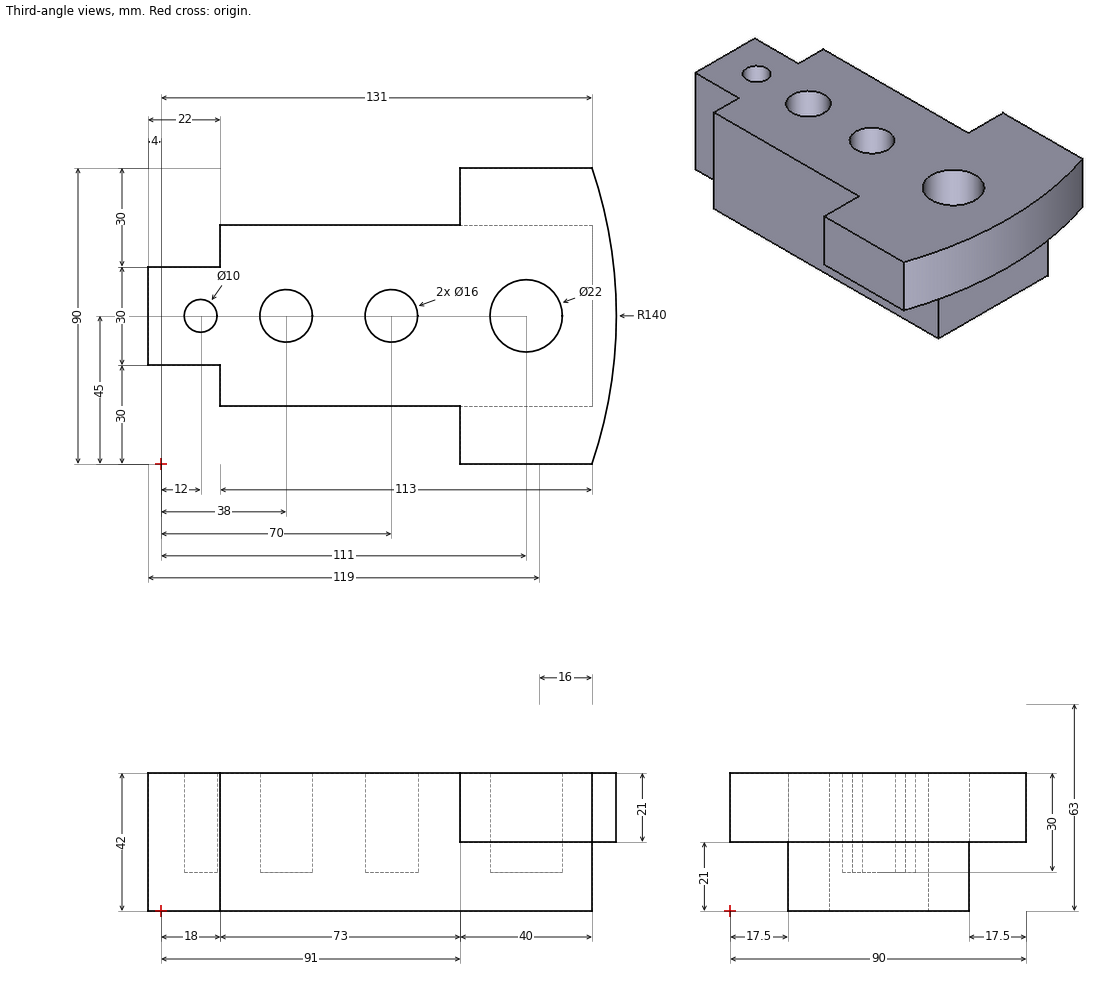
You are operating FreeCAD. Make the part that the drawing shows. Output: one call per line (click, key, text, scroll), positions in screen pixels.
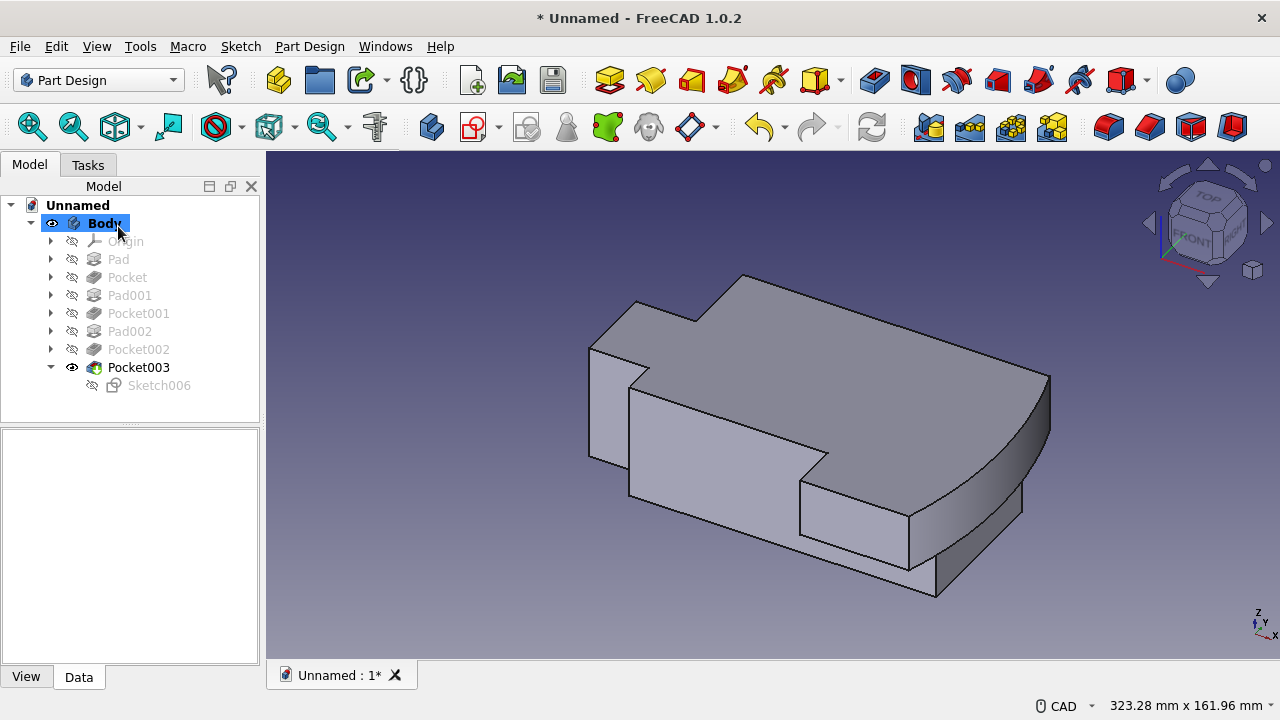
key(4)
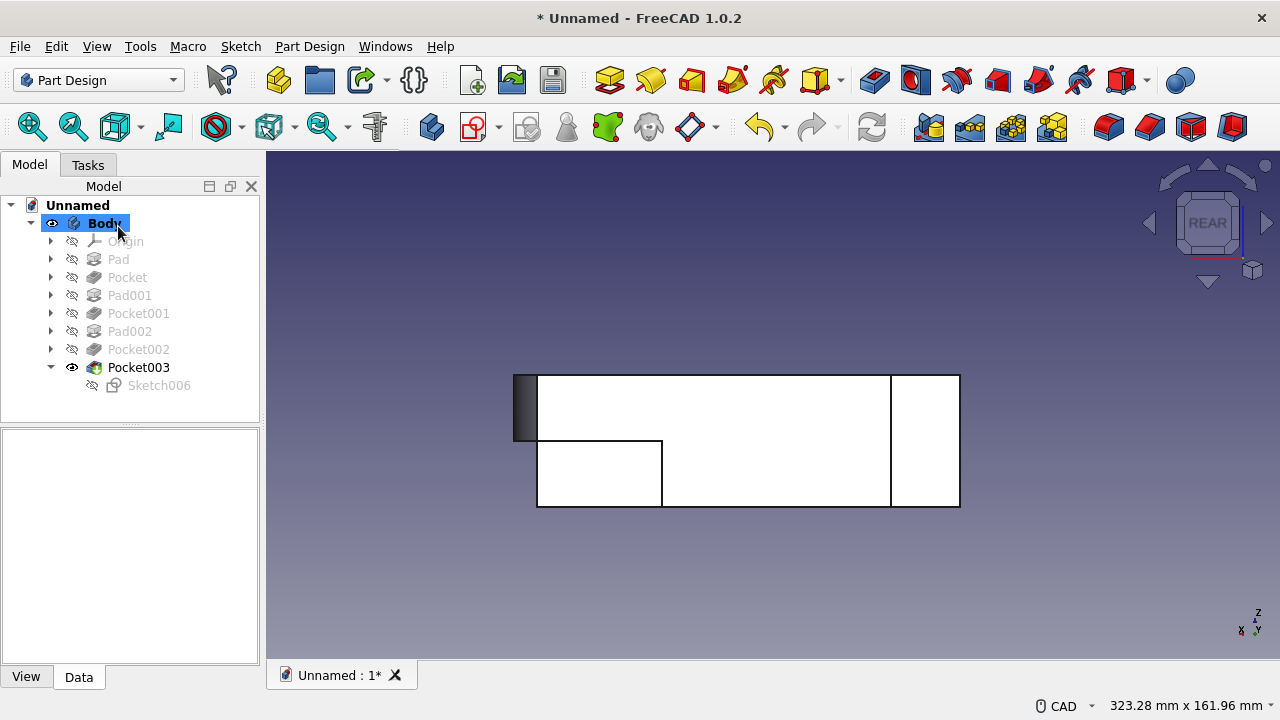
click(33, 128)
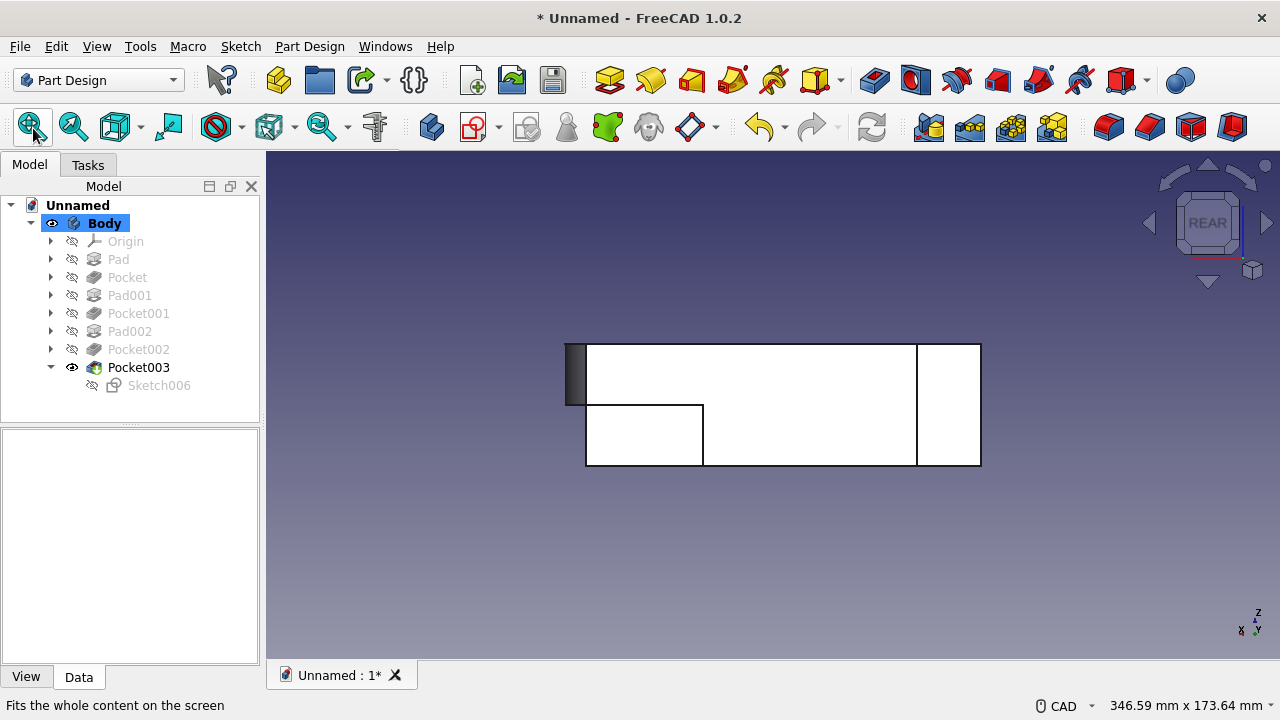
click(799, 404)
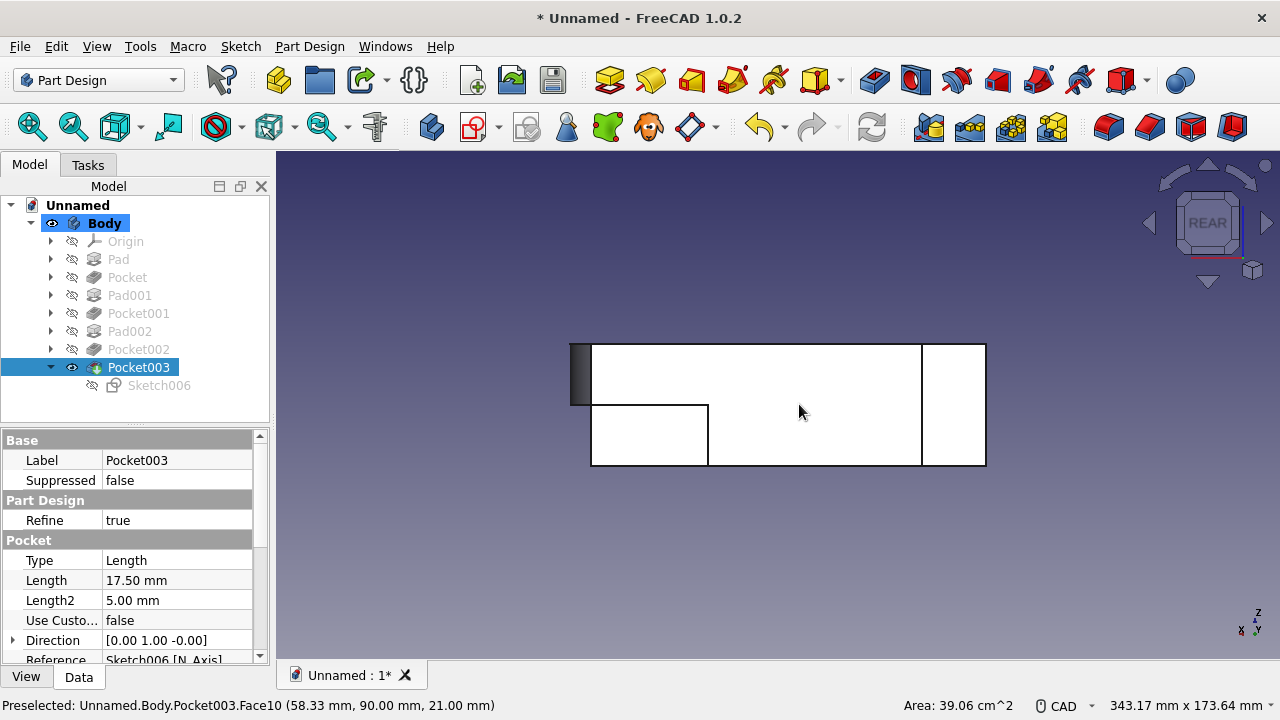
click(472, 128)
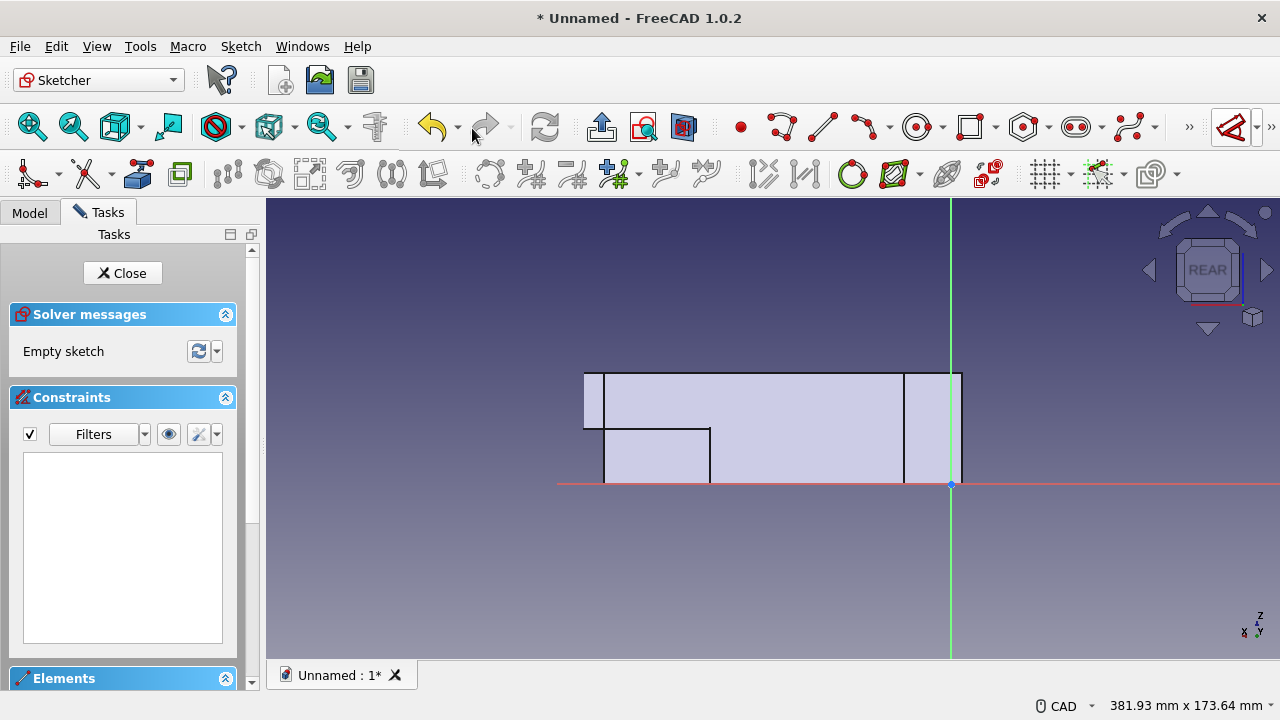
scroll(934, 428, up, 4)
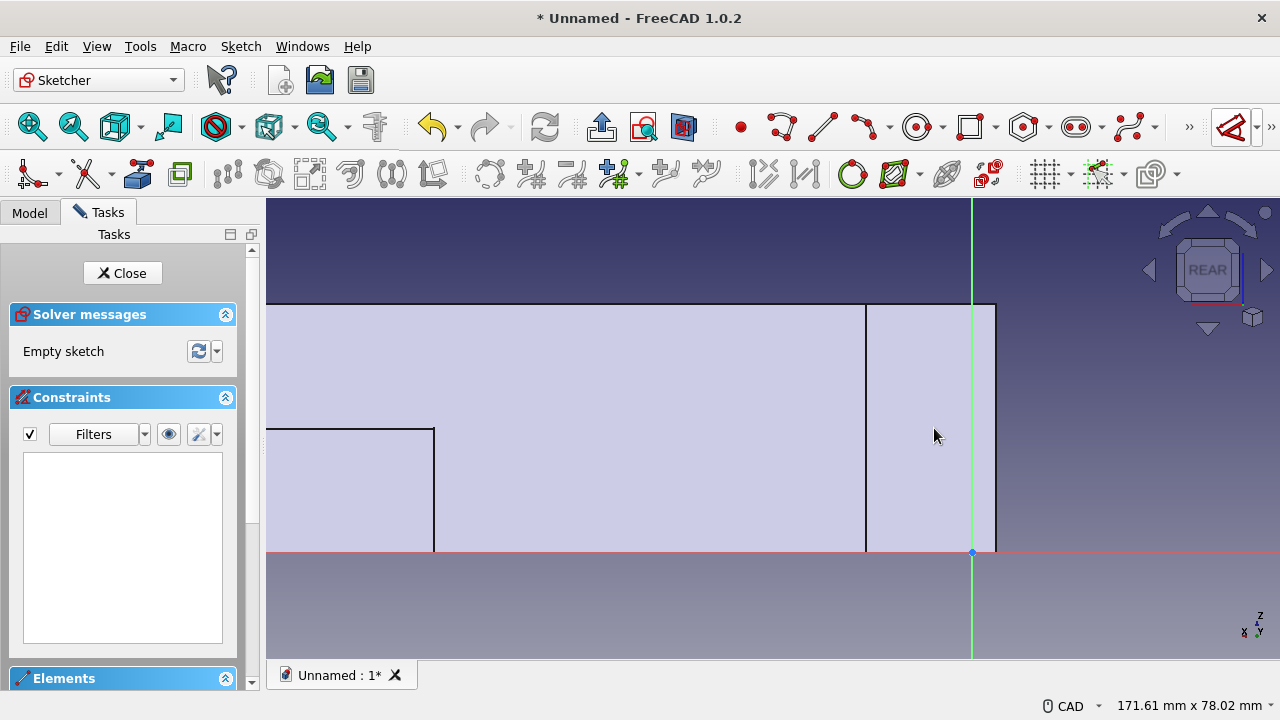
click(970, 128)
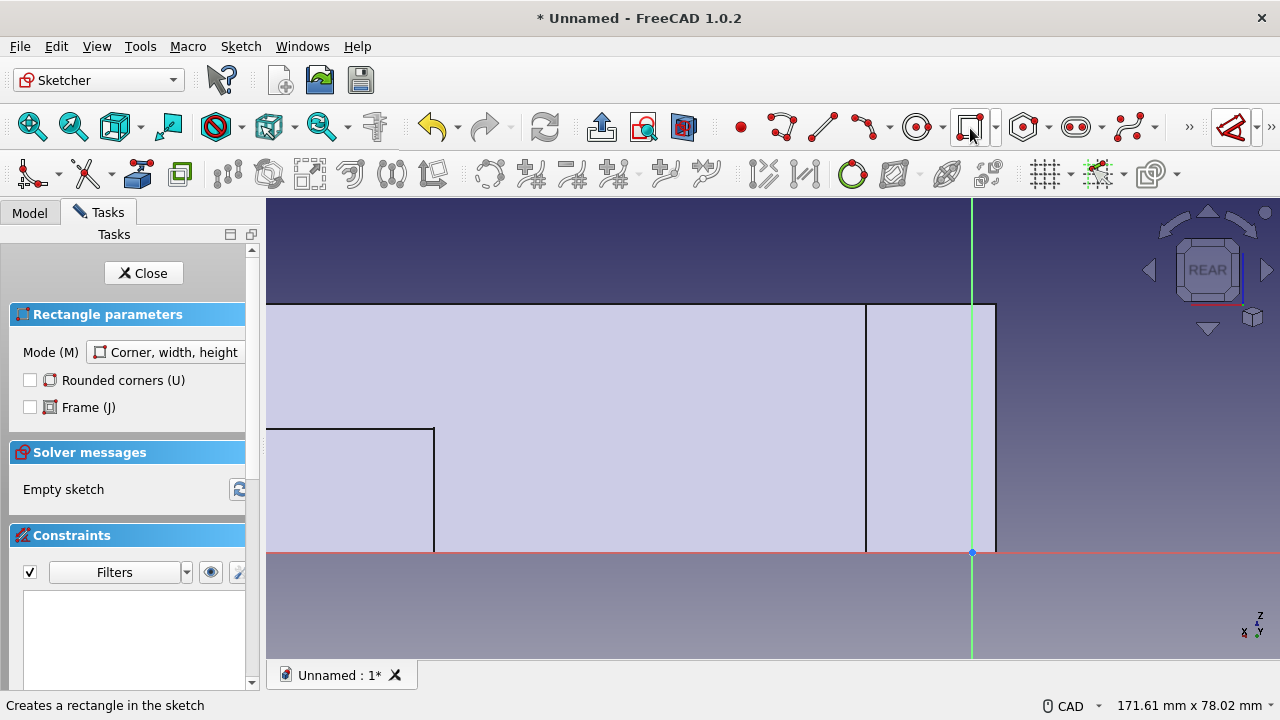
click(434, 304)
click(866, 553)
key(Escape)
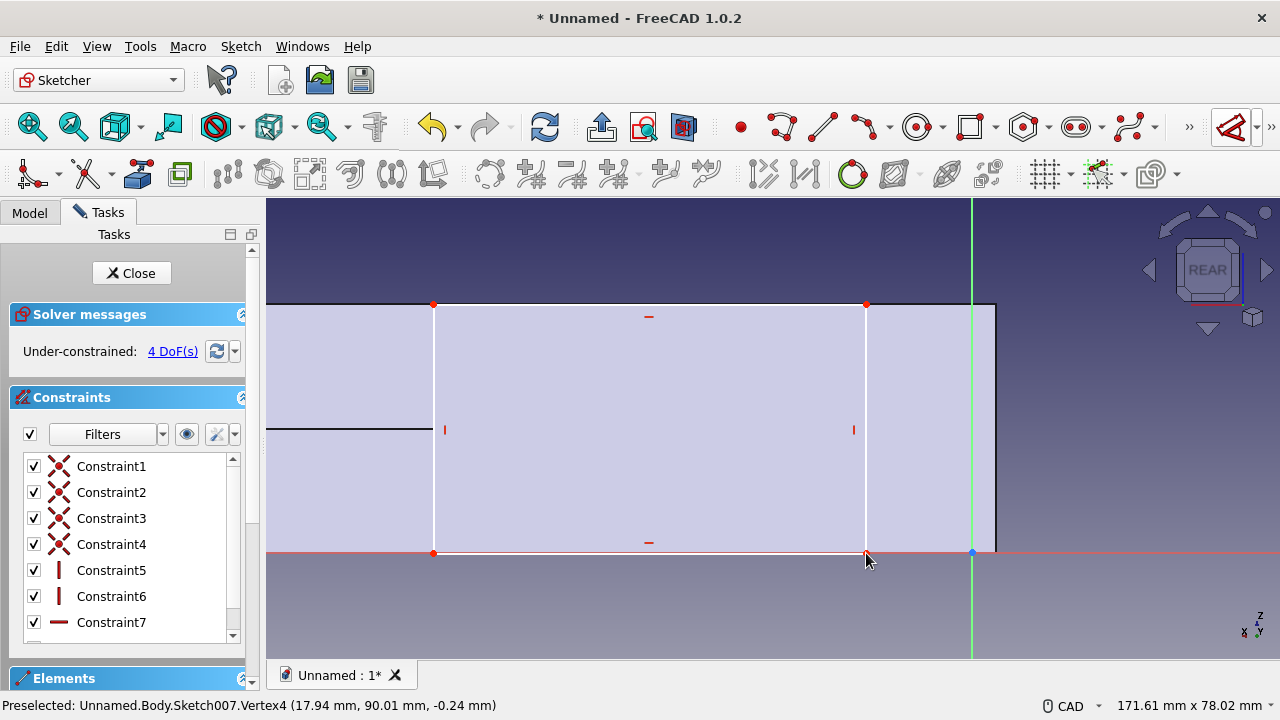
click(434, 554)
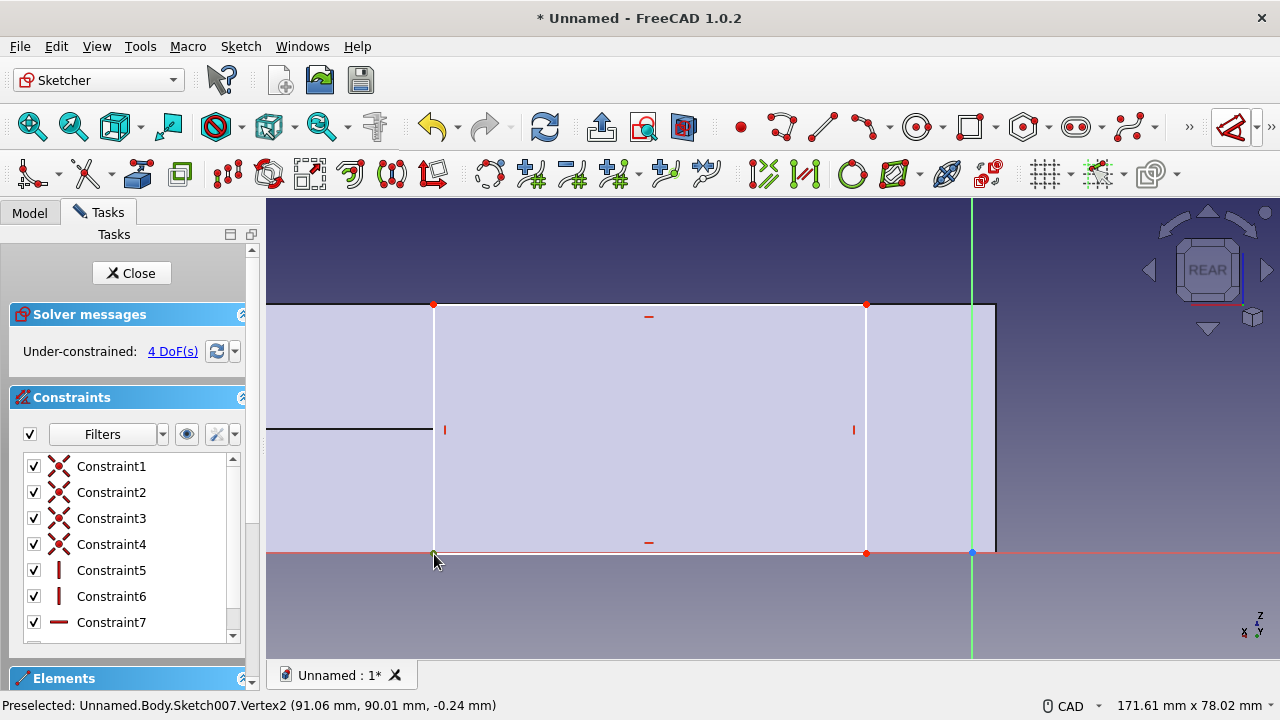
click(353, 553)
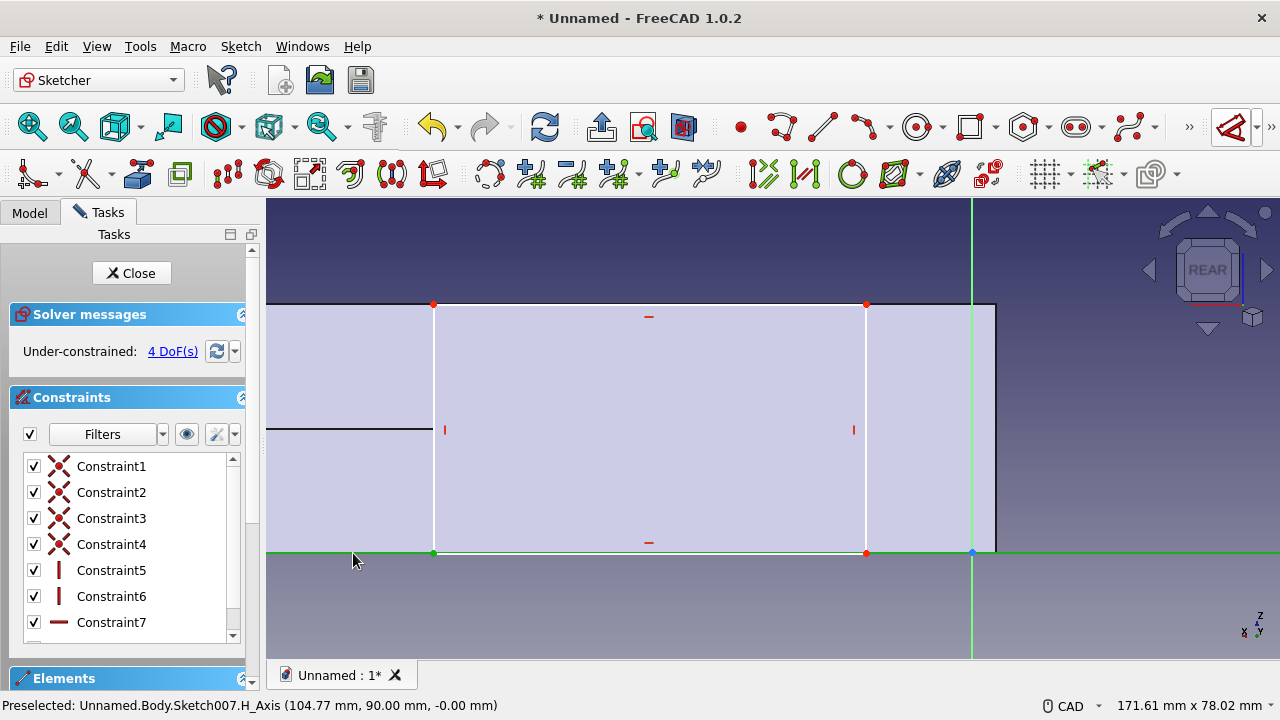
key(c)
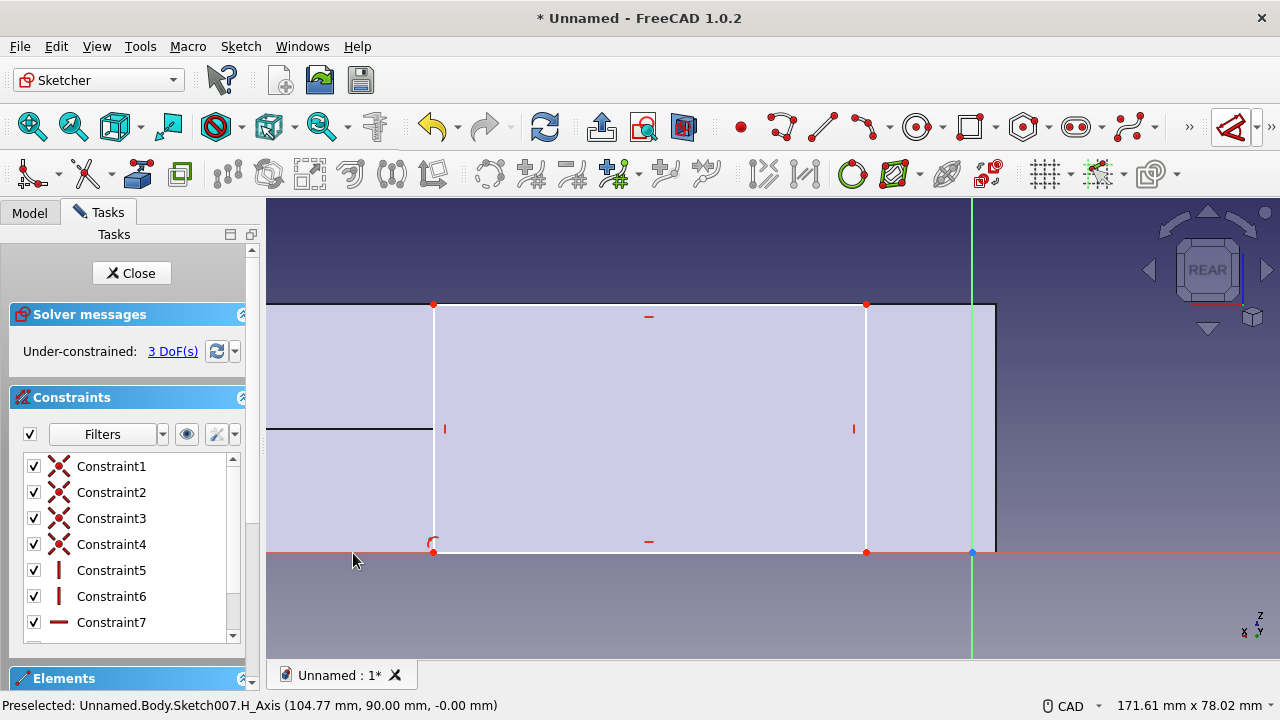
click(434, 379)